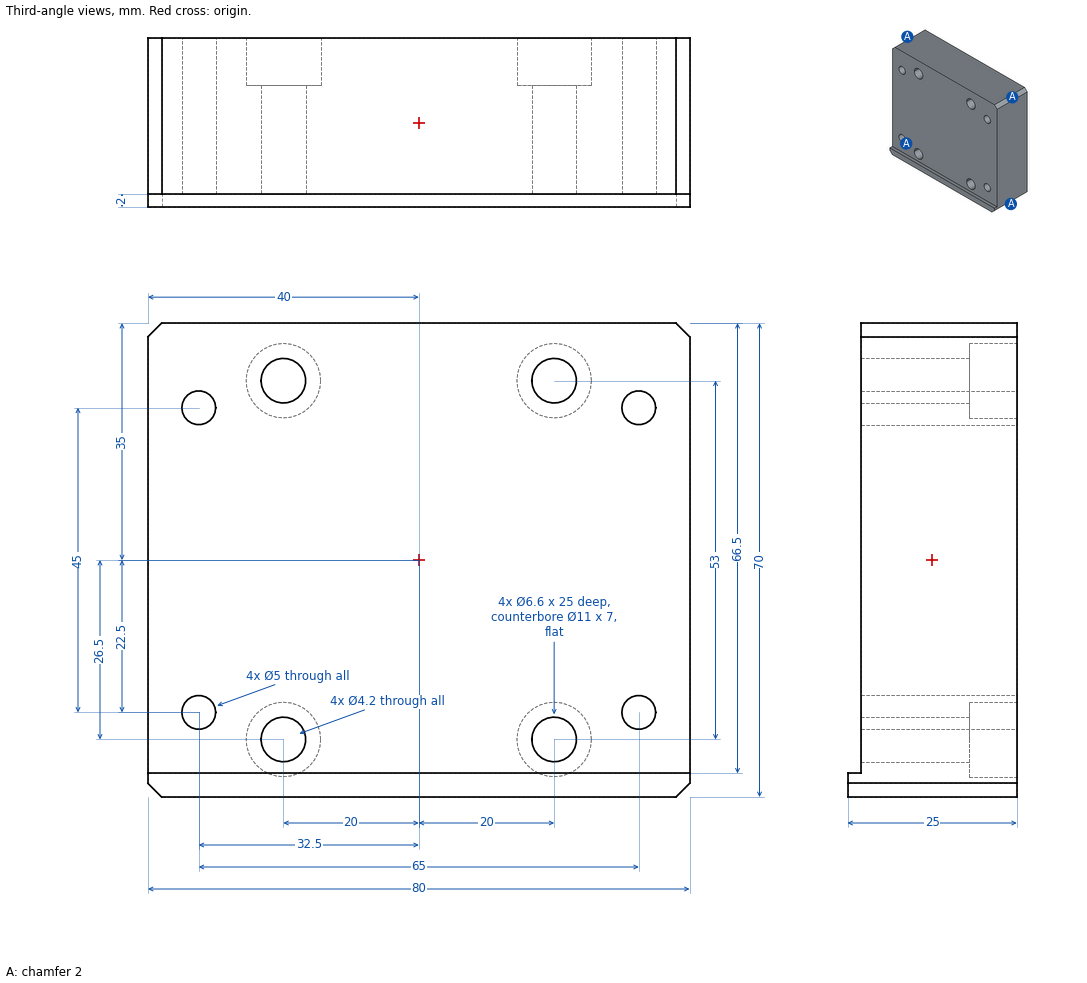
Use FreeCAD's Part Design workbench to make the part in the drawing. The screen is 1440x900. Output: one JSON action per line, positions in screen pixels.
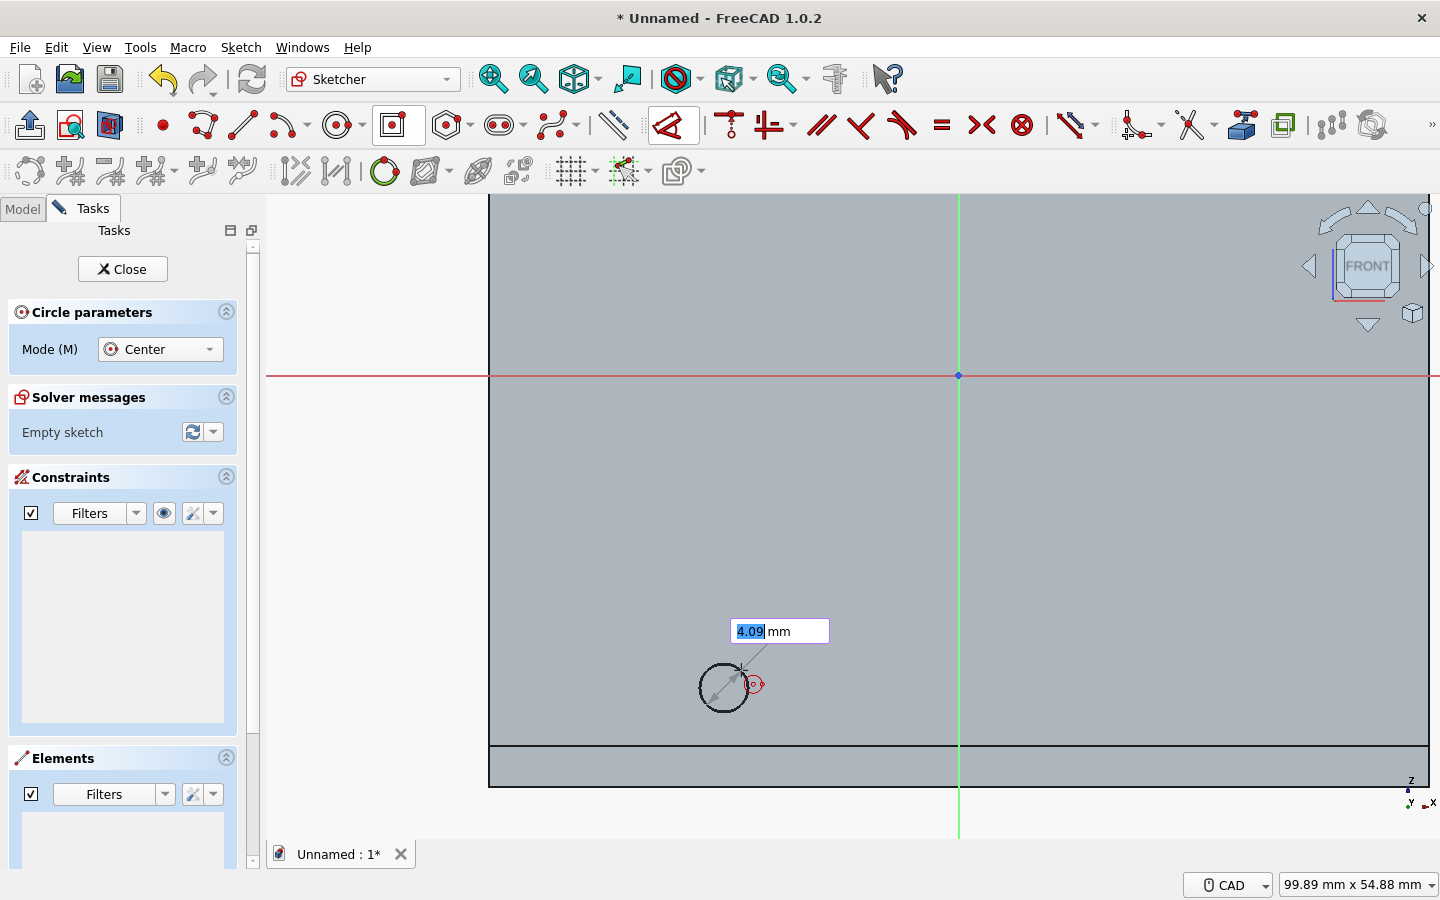
{"action": "type", "text": "4.2"}
{"action": "key", "text": "Return"}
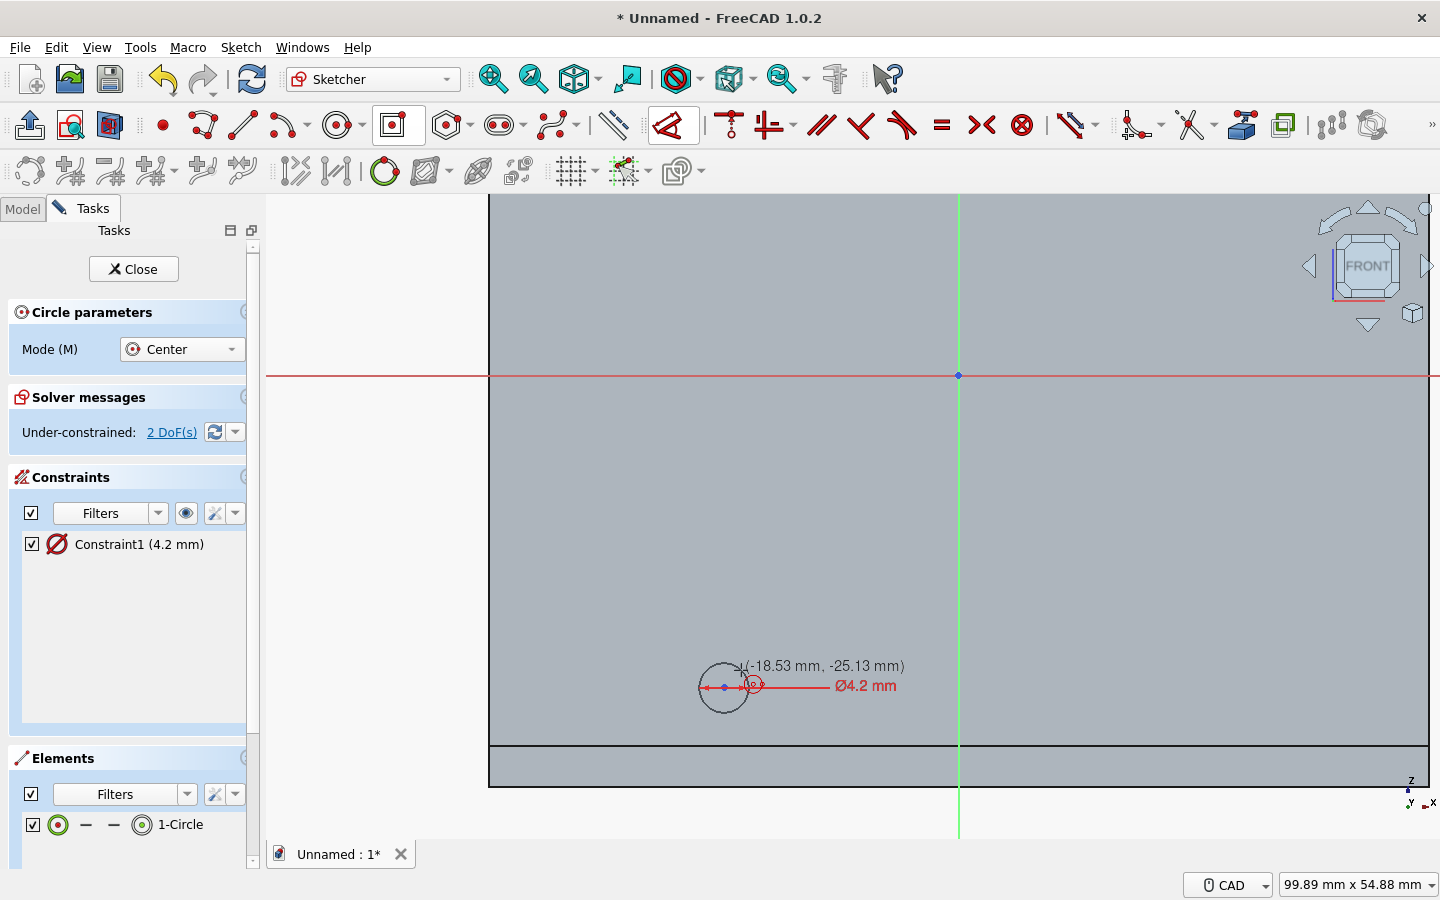
{"action": "left_click", "coordinate": [1194, 687]}
{"action": "mouse_move", "coordinate": [1211, 670]}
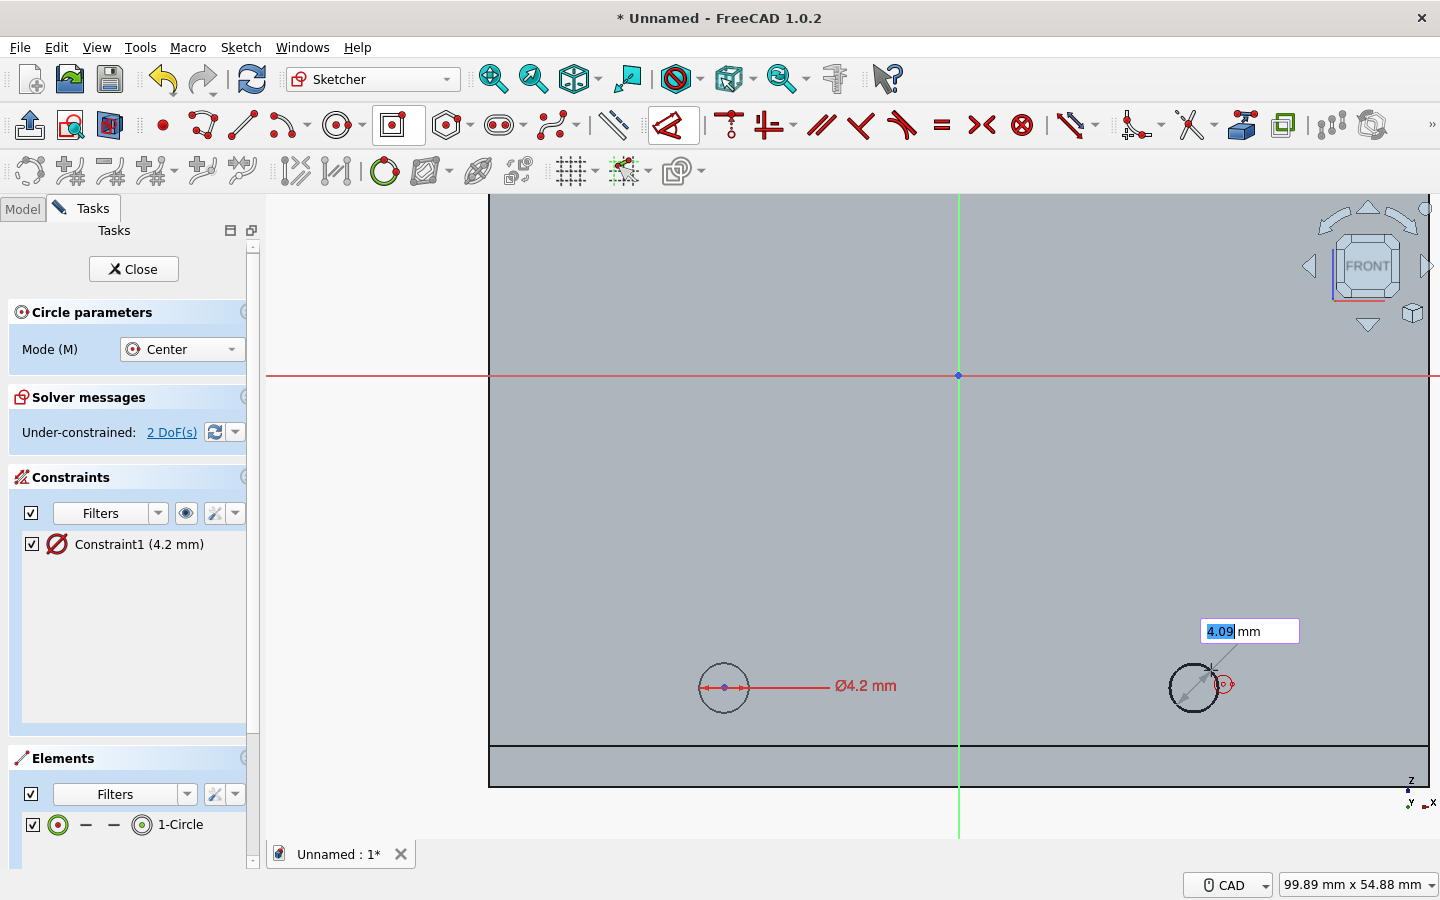
{"action": "type", "text": "4.2"}
{"action": "key", "text": "Return"}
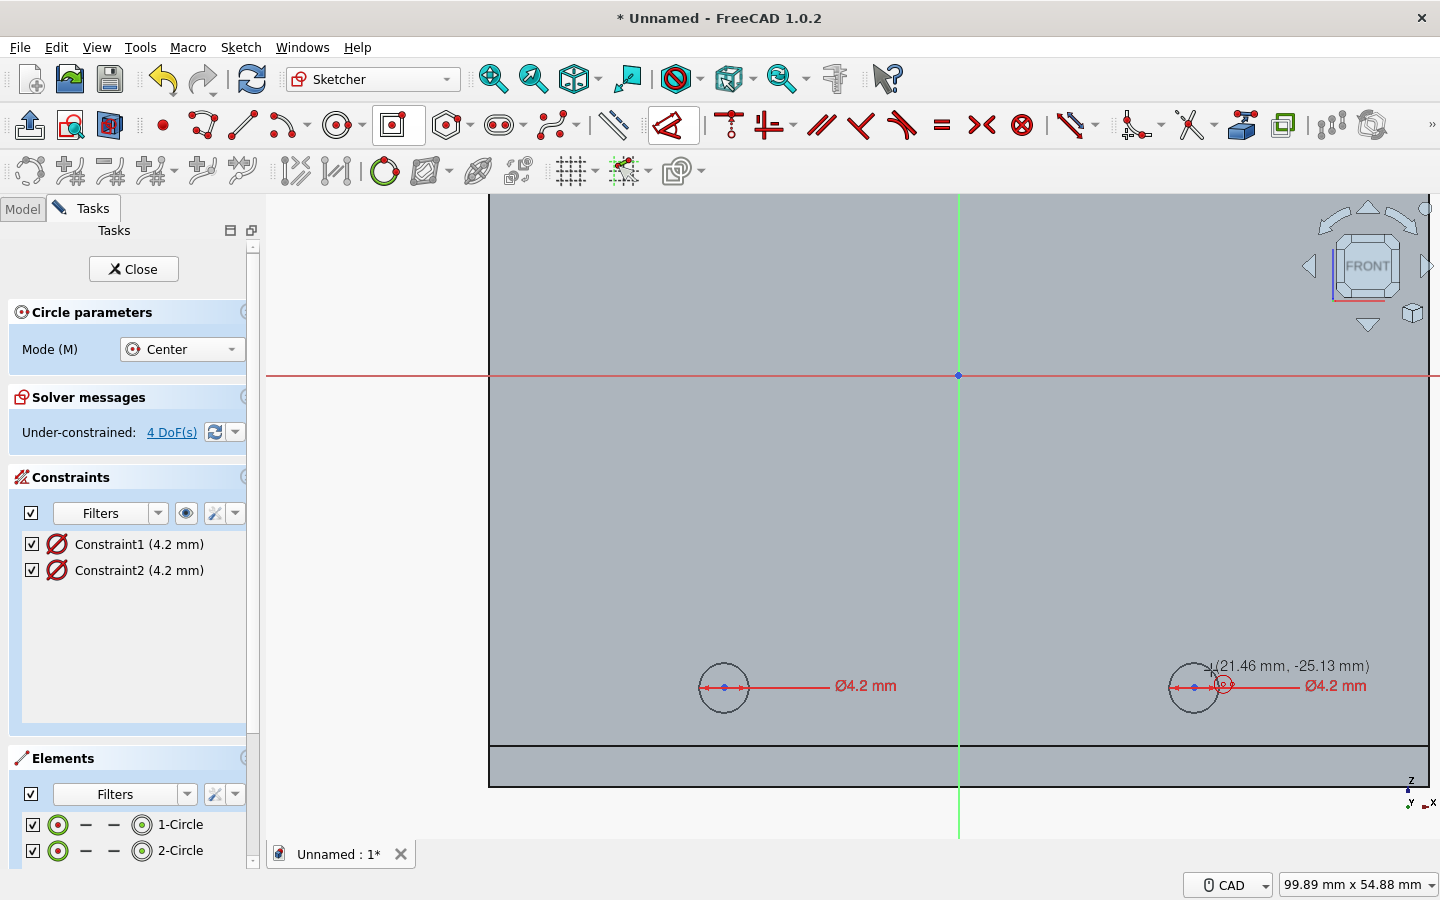
{"action": "scroll", "coordinate": [430, 803], "scroll_direction": "down", "scroll_amount": 2}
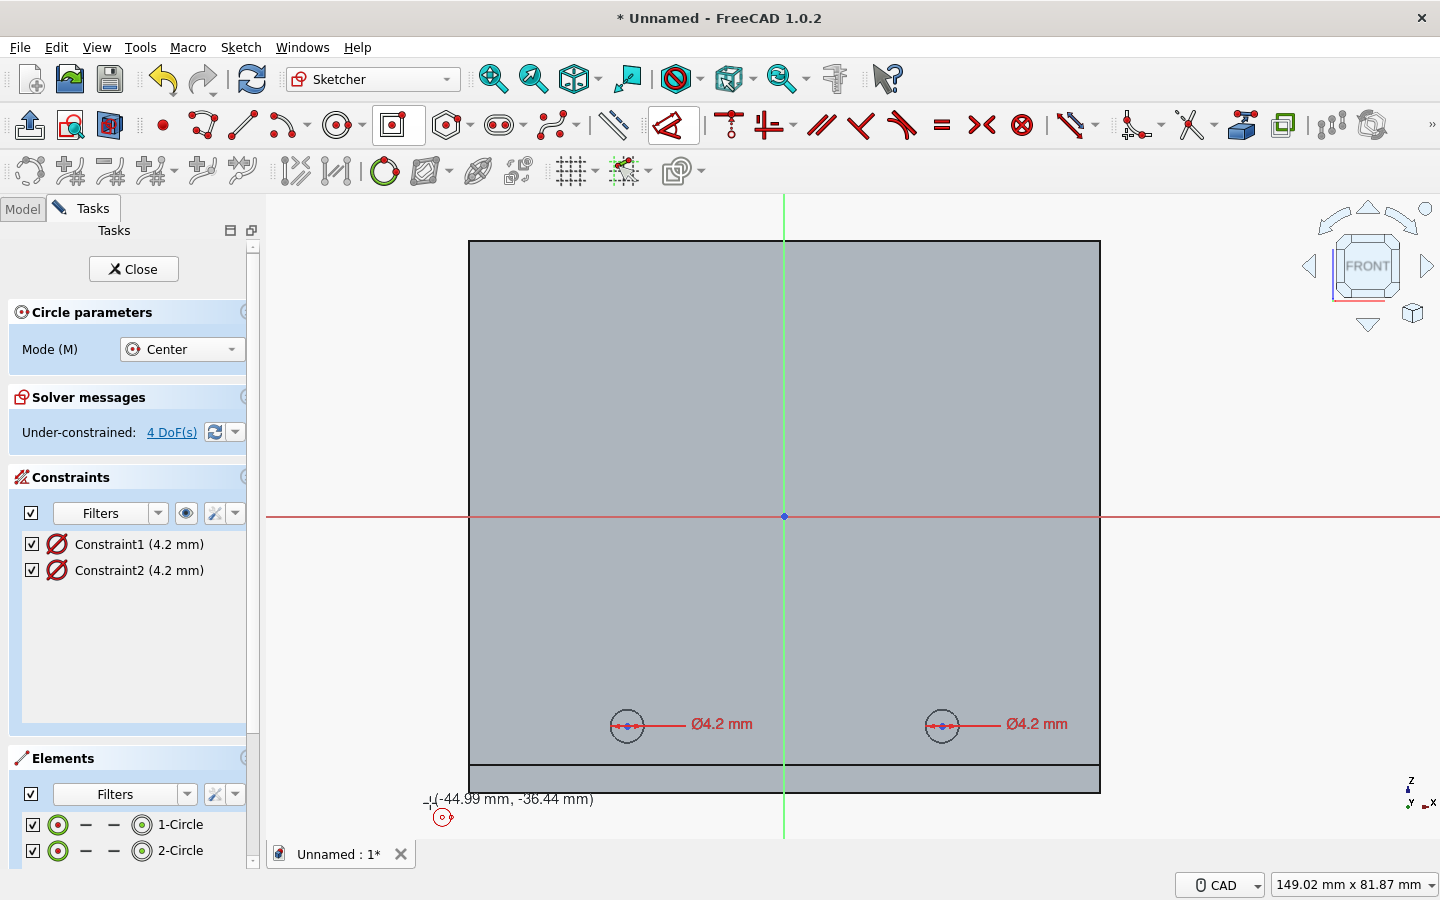
{"action": "scroll", "coordinate": [942, 308], "scroll_direction": "up", "scroll_amount": 2}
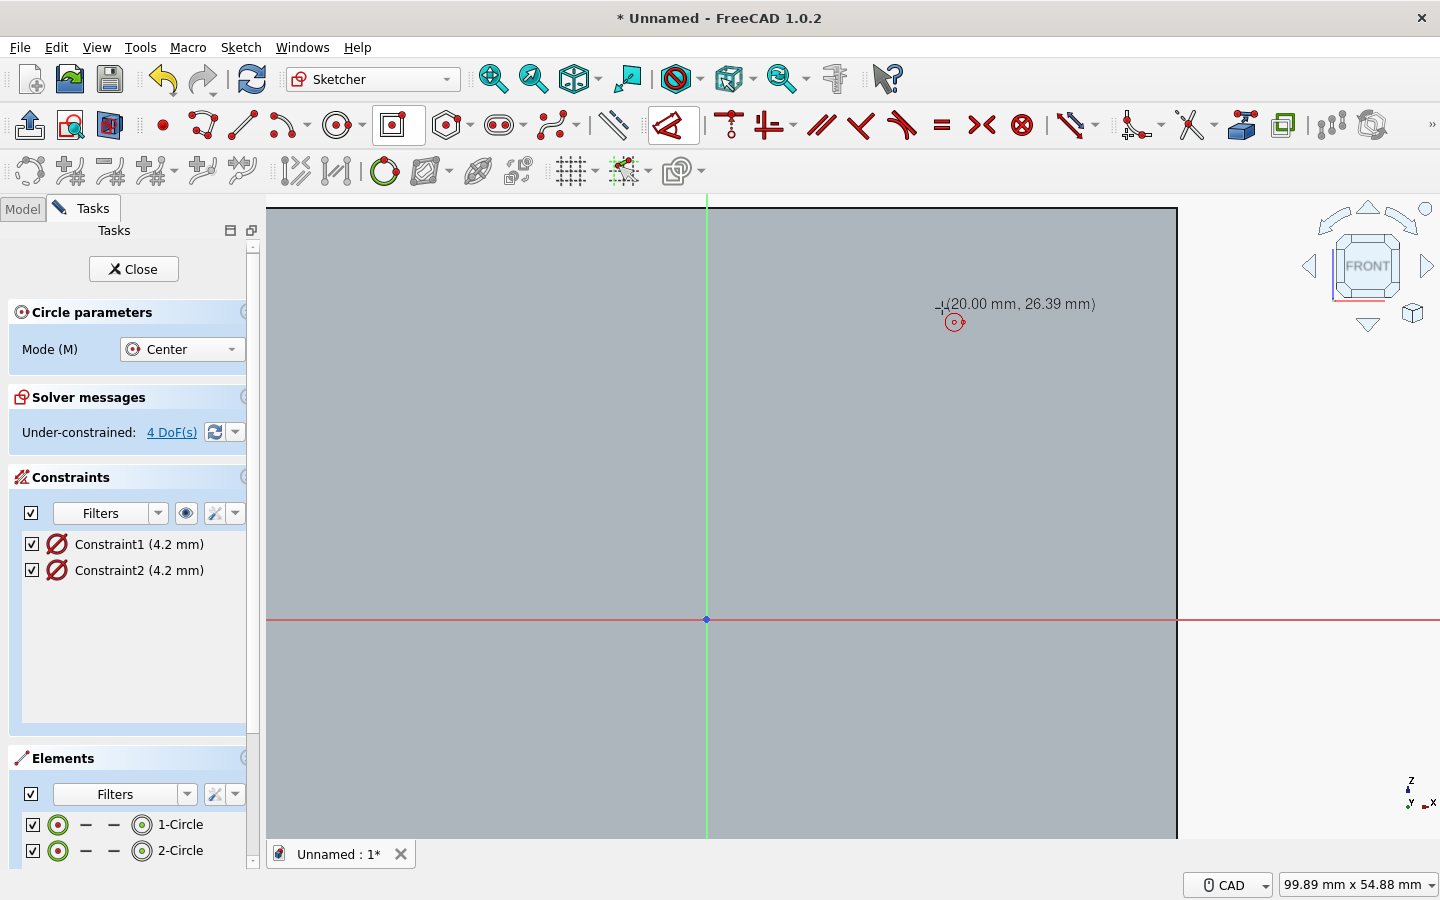
{"action": "left_click", "coordinate": [942, 308]}
{"action": "mouse_move", "coordinate": [959, 291]}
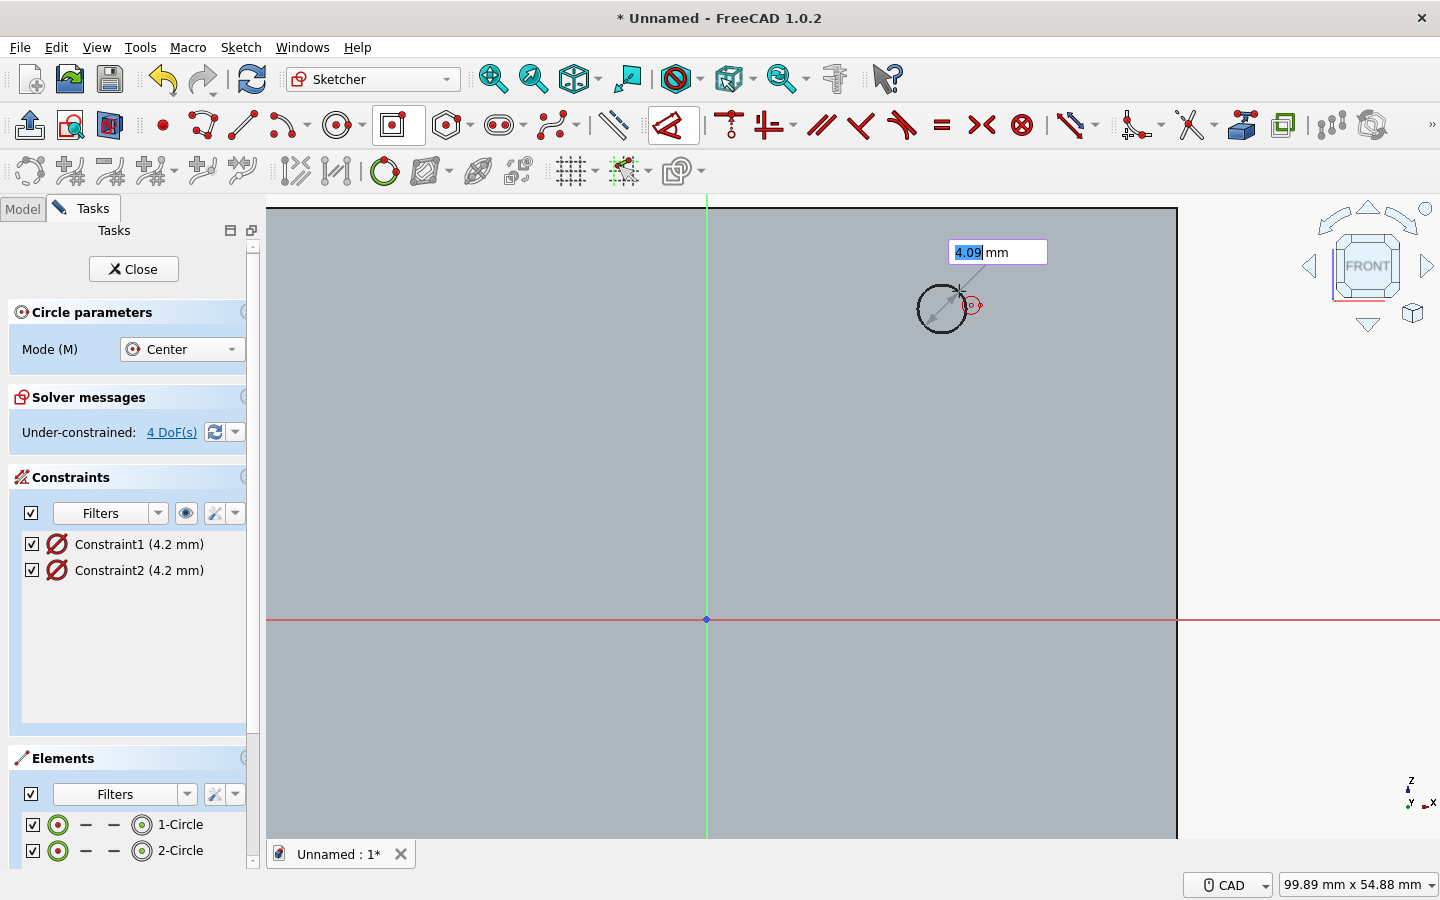
{"action": "type", "text": "4.2"}
{"action": "key", "text": "Return"}